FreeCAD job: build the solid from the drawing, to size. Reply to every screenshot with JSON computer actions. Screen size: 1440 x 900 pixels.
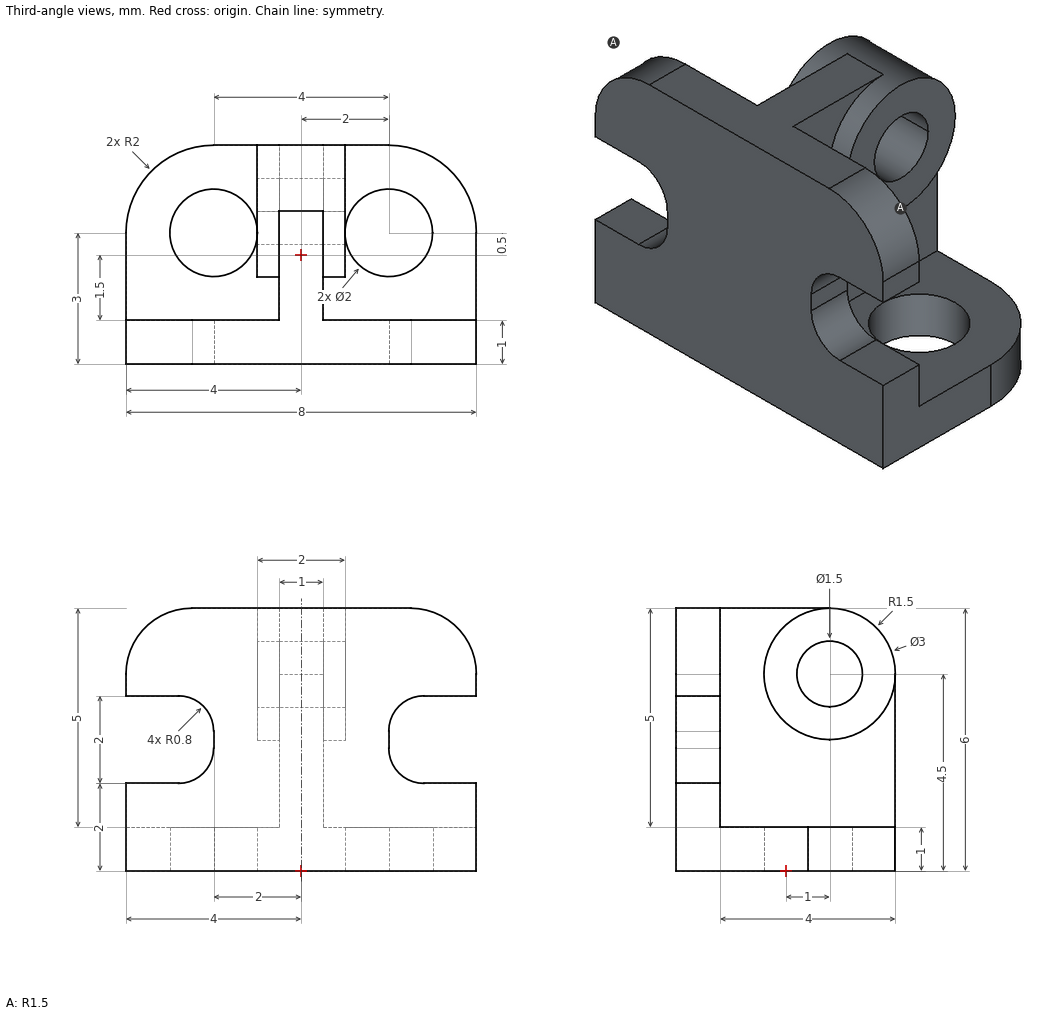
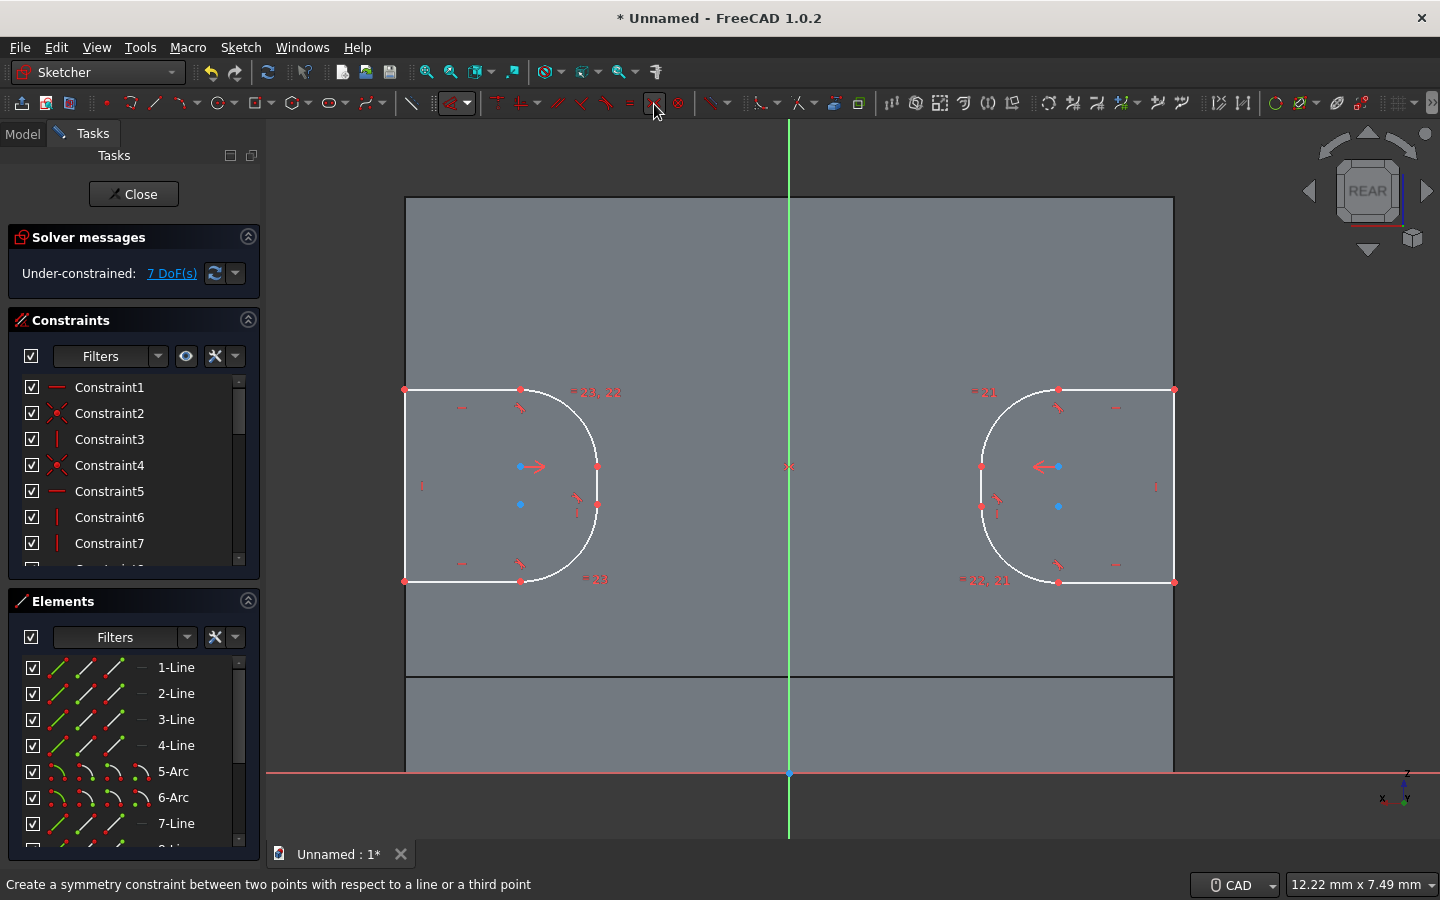
{"action": "left_click", "coordinate": [1174, 583]}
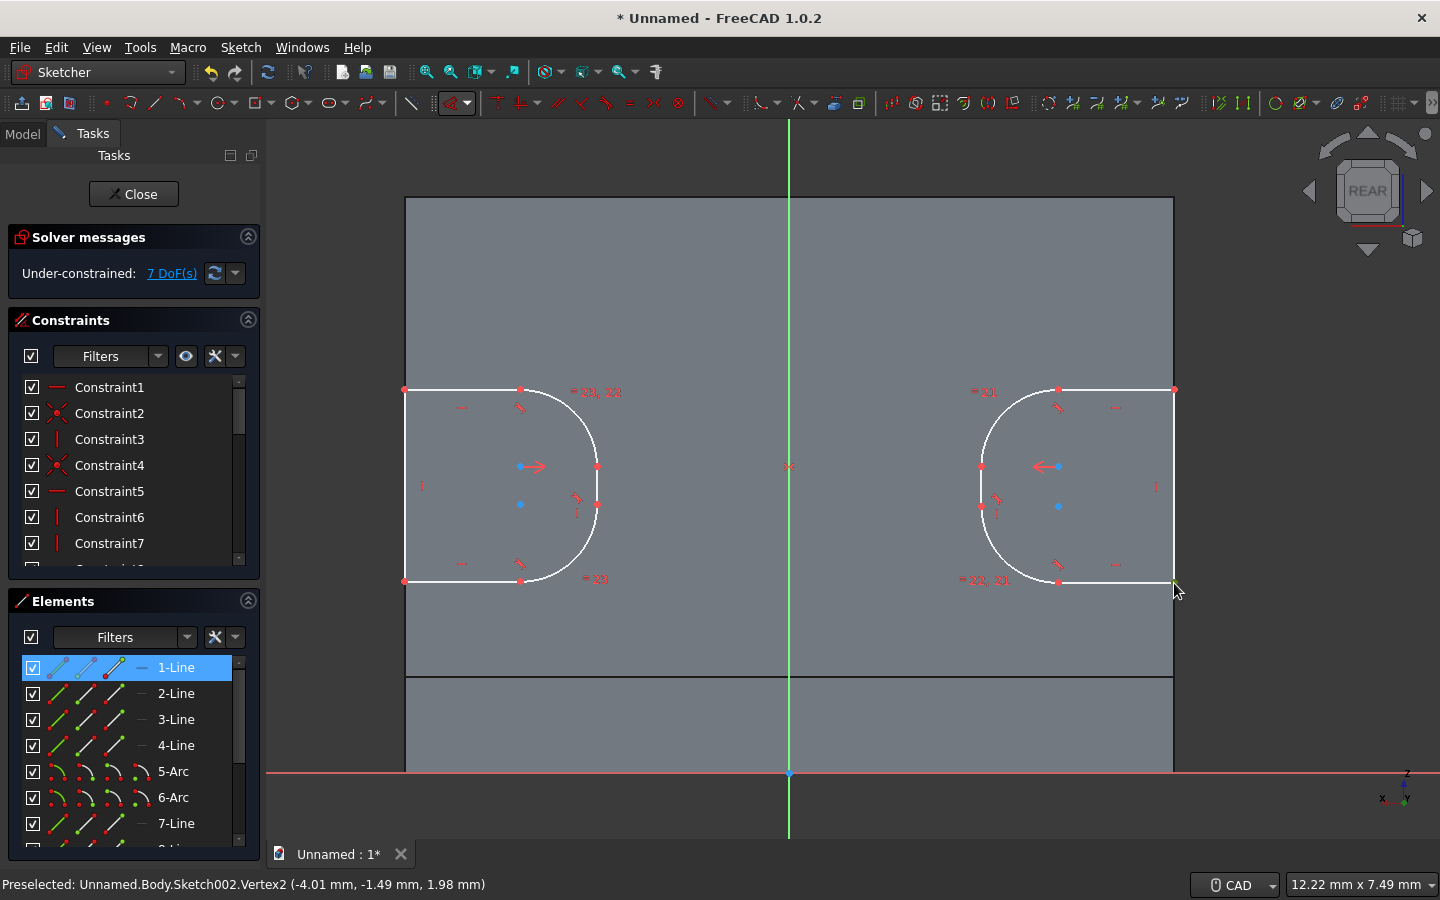
{"action": "left_click", "coordinate": [405, 582]}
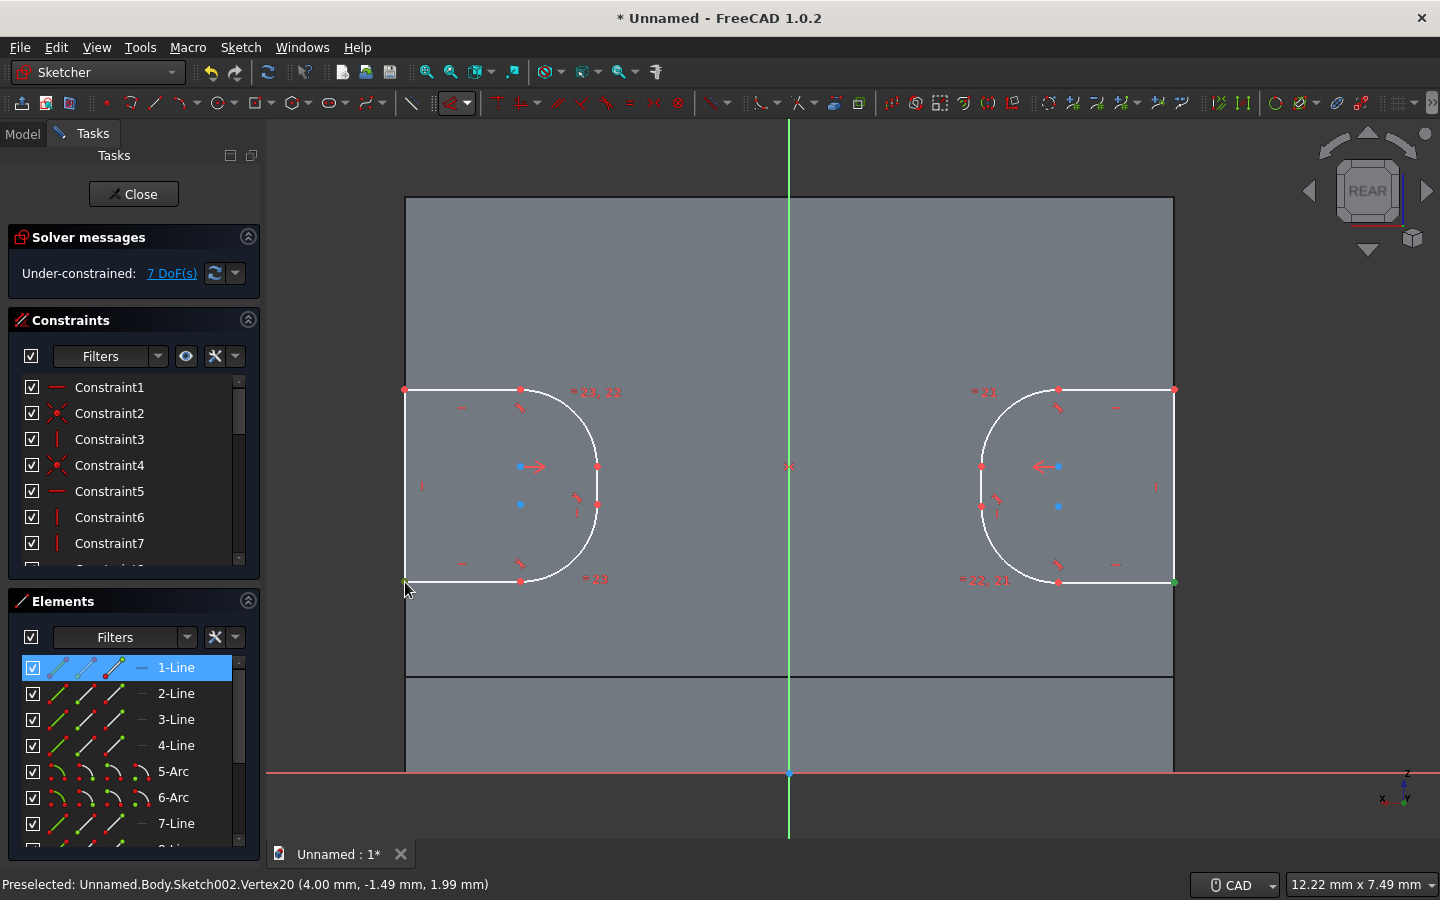
{"action": "left_click", "coordinate": [789, 716]}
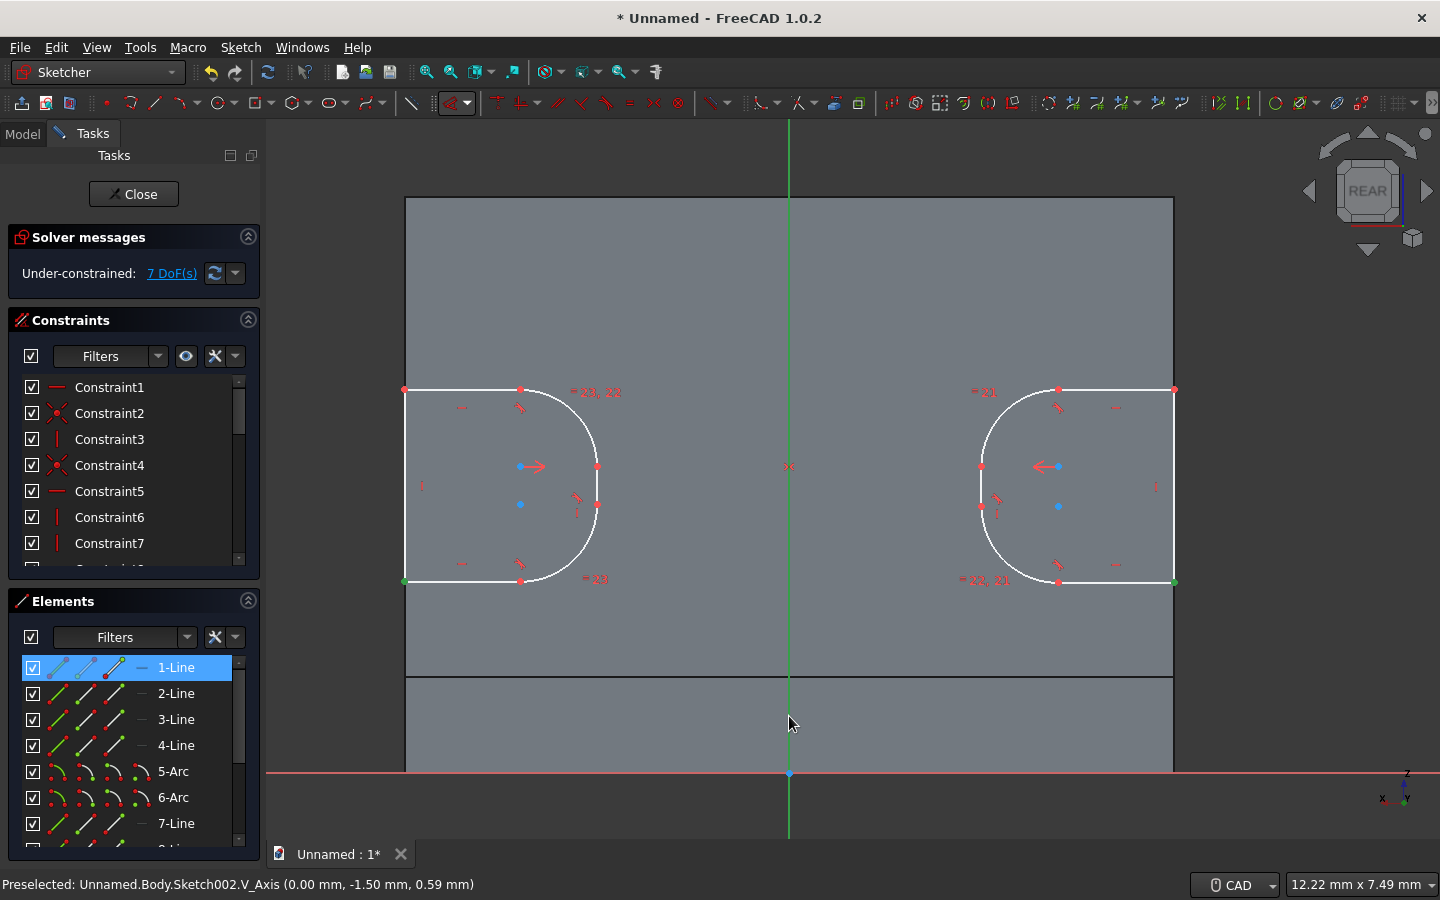
{"action": "left_click", "coordinate": [654, 104]}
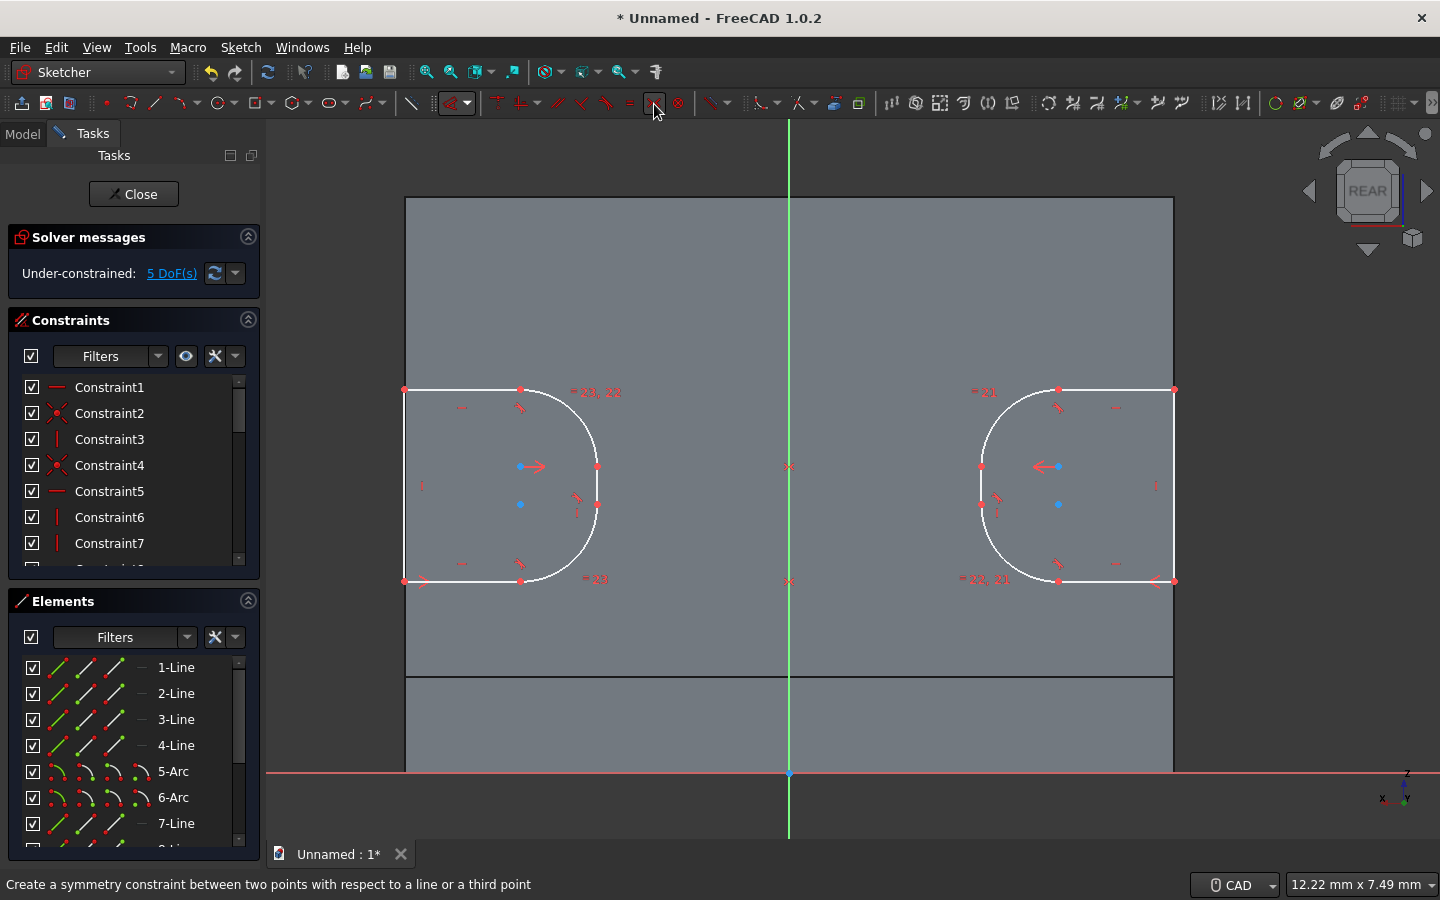
{"action": "left_click", "coordinate": [1023, 398]}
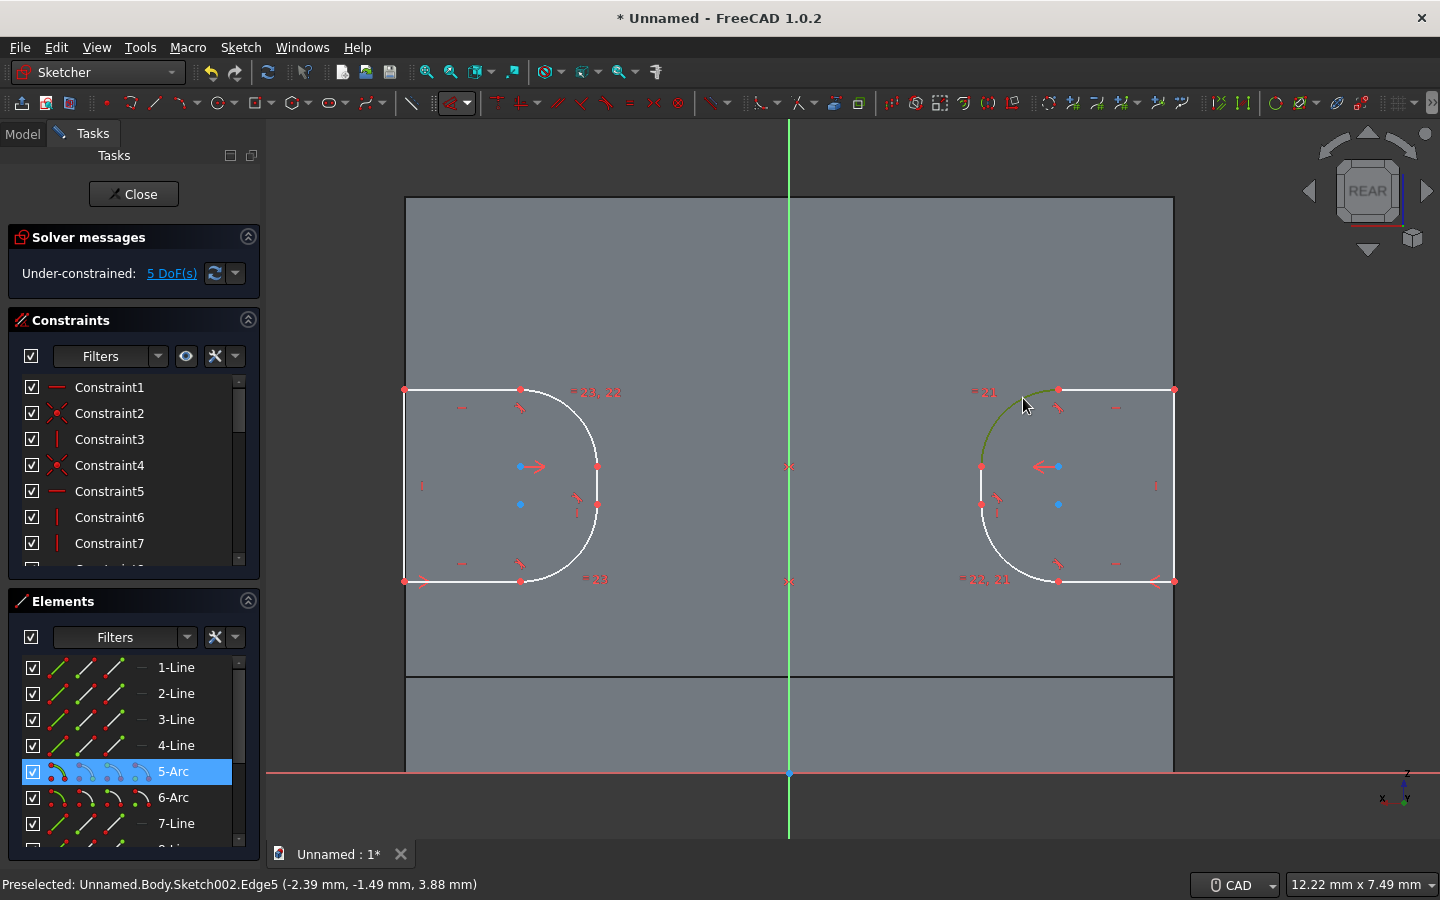
{"action": "key", "text": "k r"}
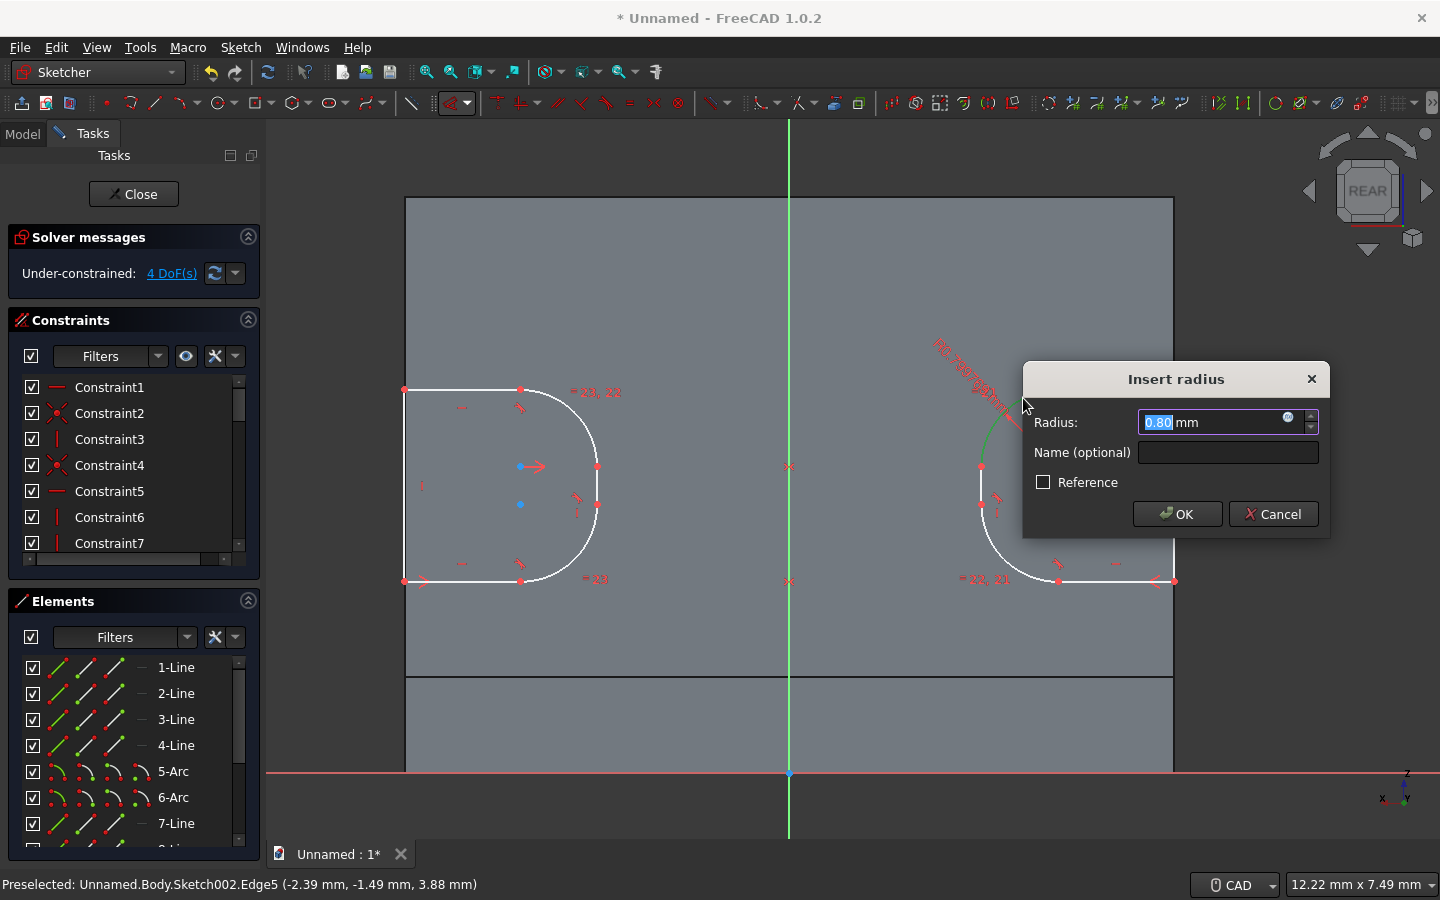
{"action": "type", "text": "0.8"}
{"action": "key", "text": "Return"}